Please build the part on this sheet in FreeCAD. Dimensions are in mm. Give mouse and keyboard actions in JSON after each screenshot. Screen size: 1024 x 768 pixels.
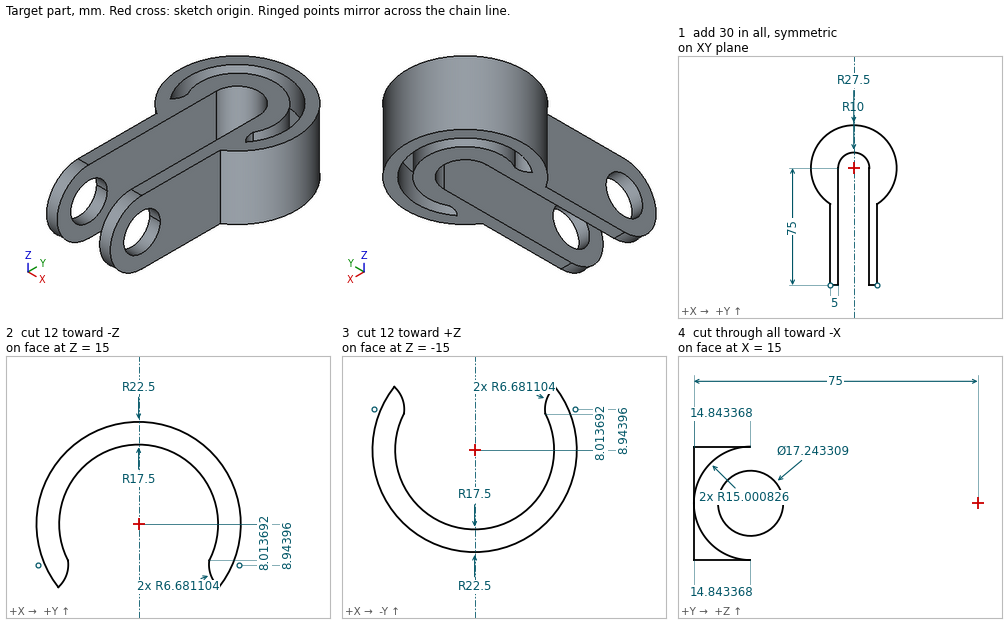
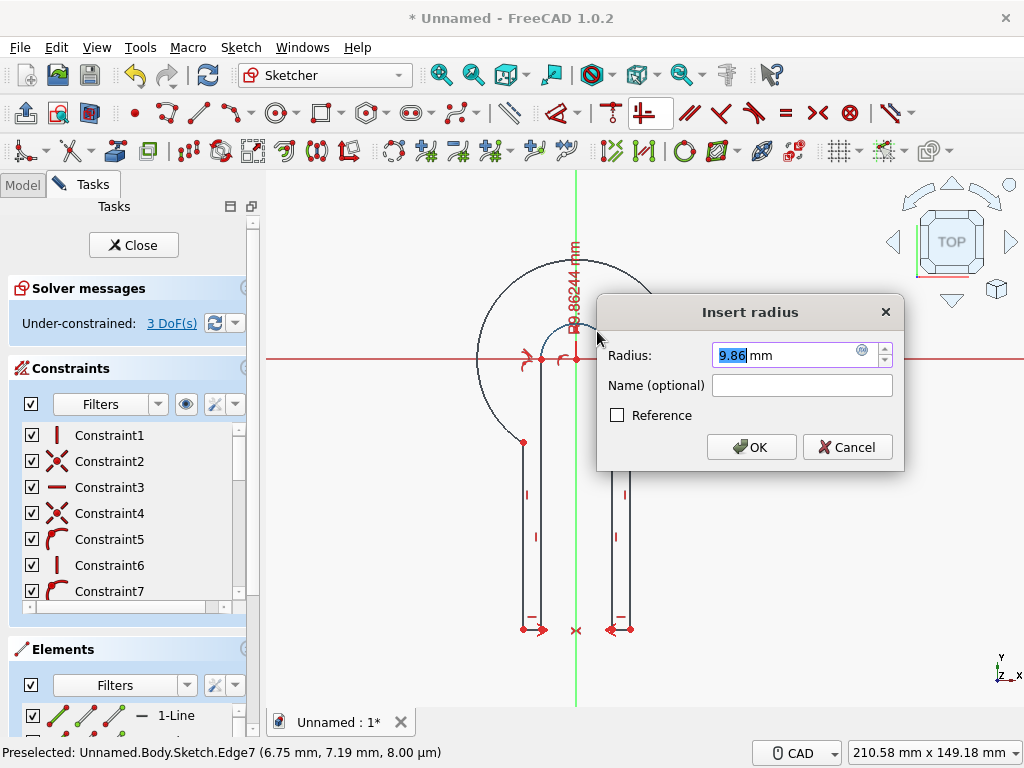
{"action": "type", "text": "10"}
{"action": "key", "text": "Return"}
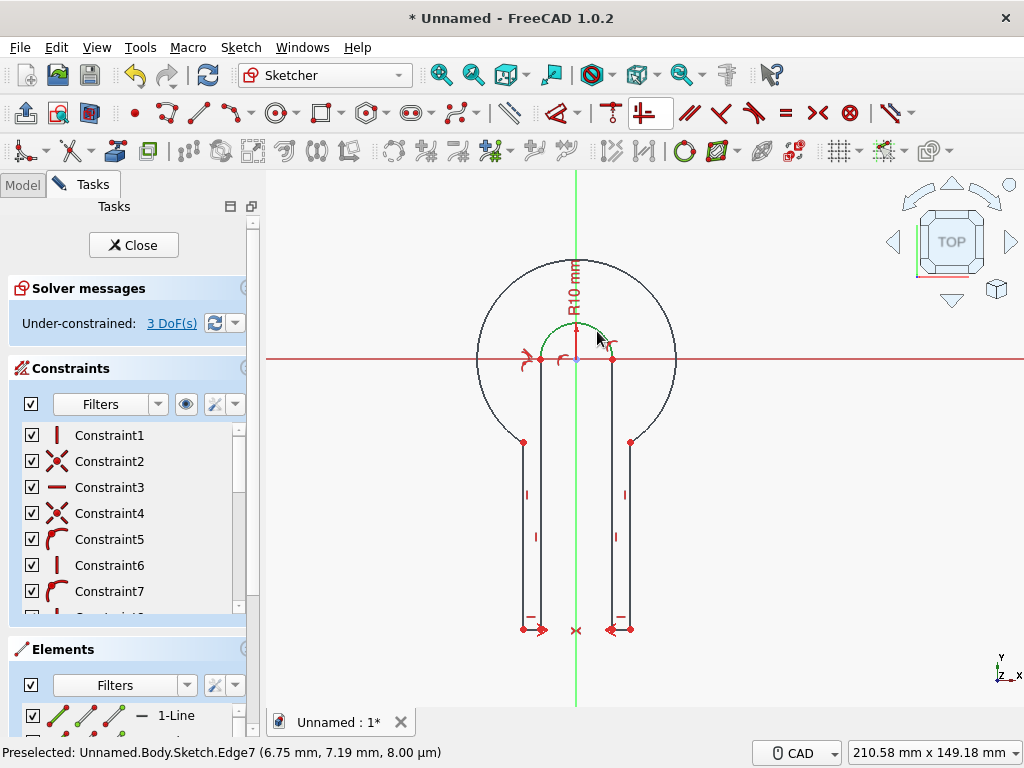
{"action": "left_click", "coordinate": [662, 308]}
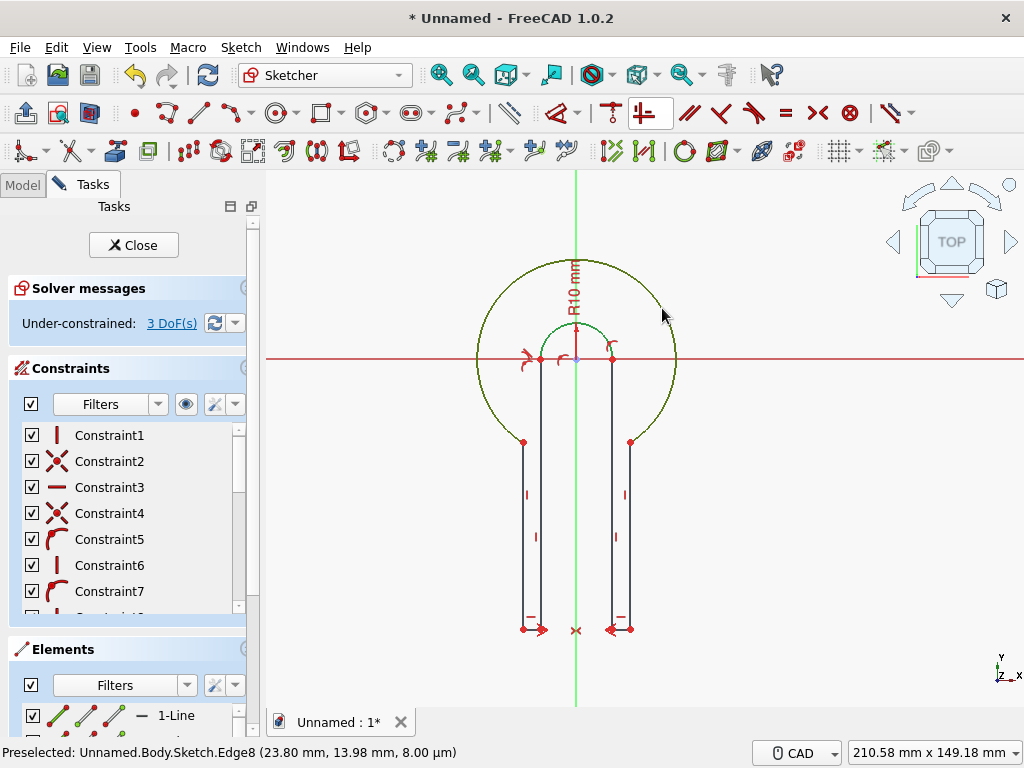
{"action": "key", "text": "k r"}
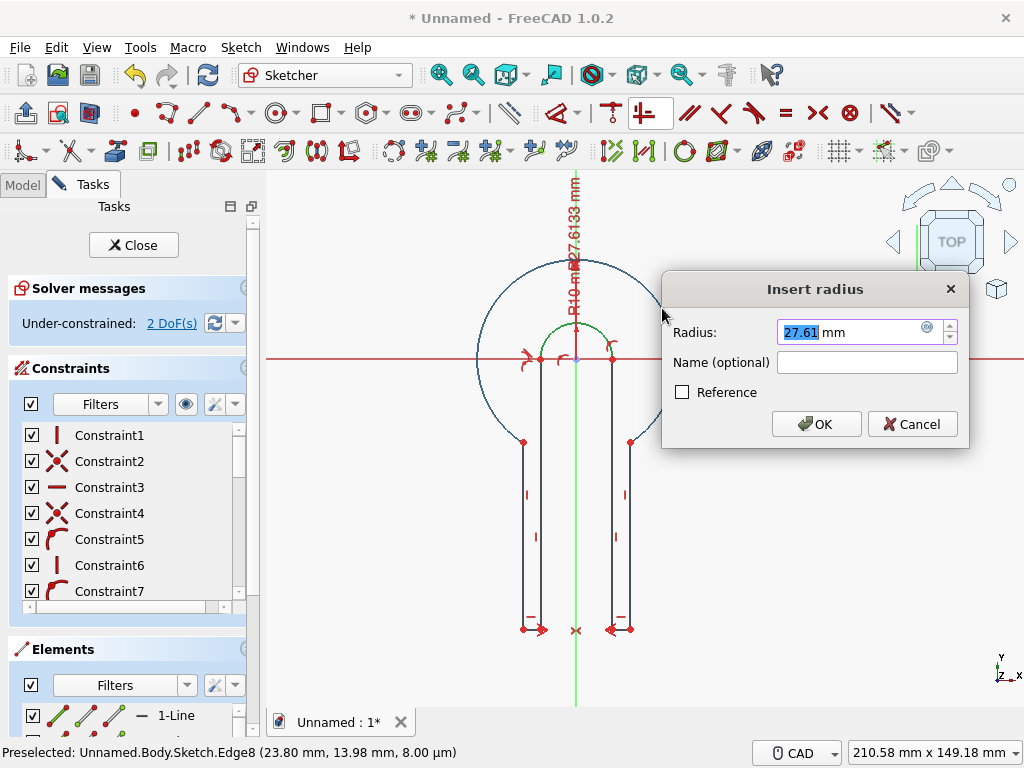
{"action": "type", "text": "27.5"}
{"action": "key", "text": "Return"}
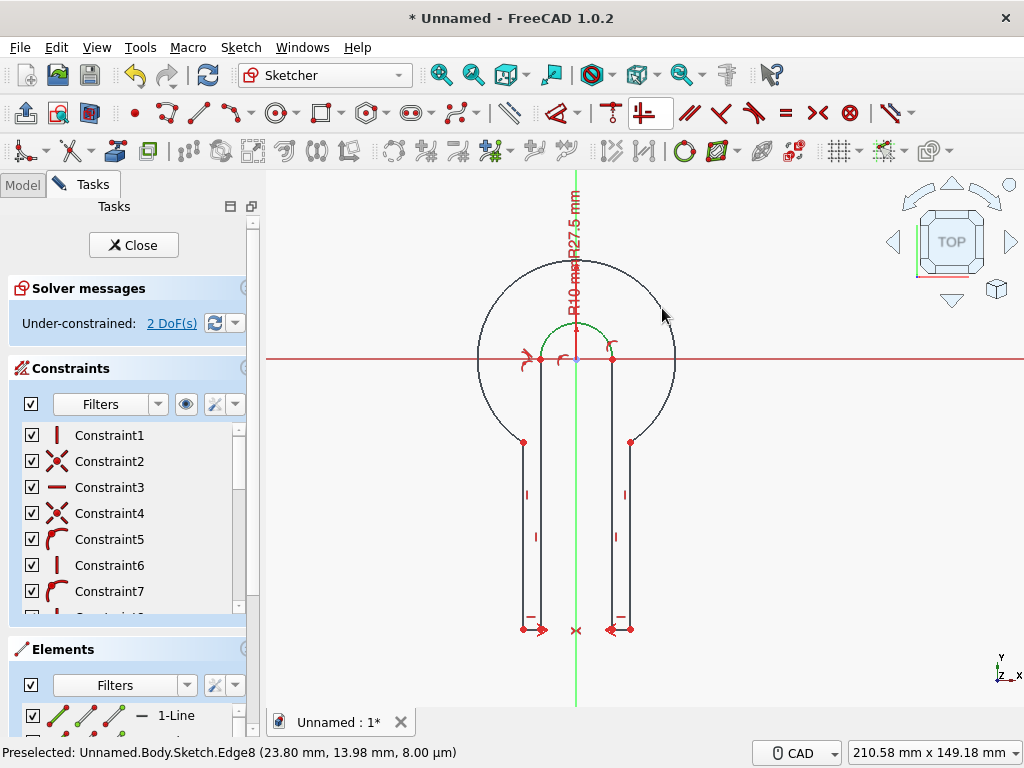
{"action": "scroll", "coordinate": [532, 630], "scroll_direction": "up", "scroll_amount": 4}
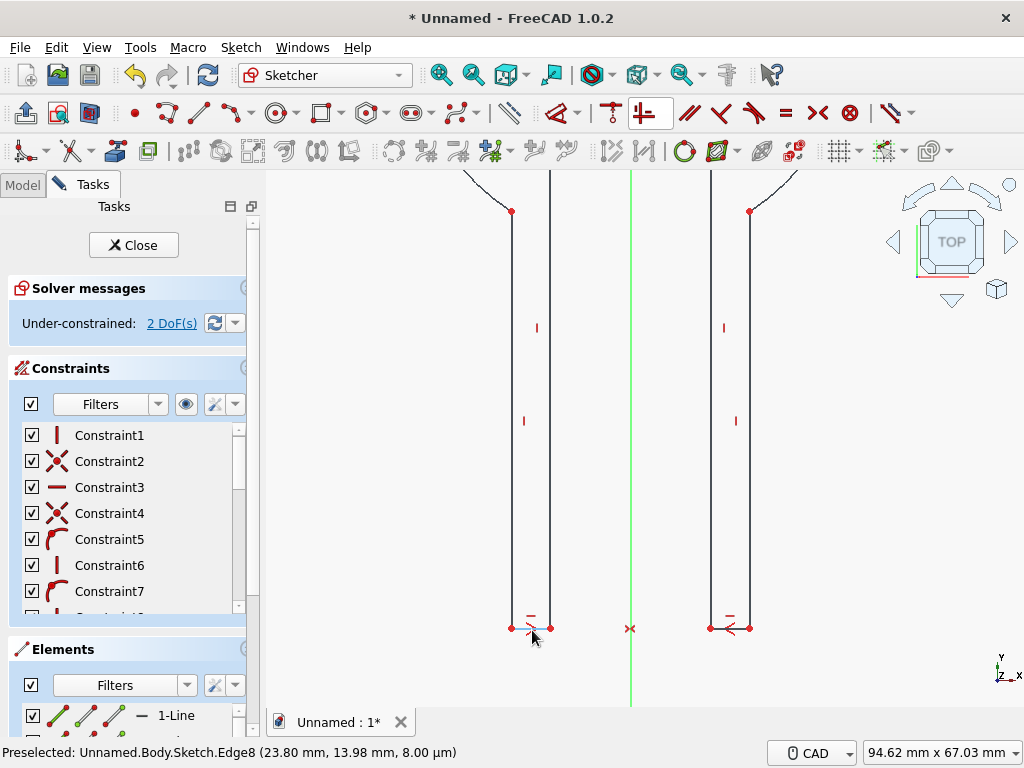
{"action": "left_click", "coordinate": [531, 629]}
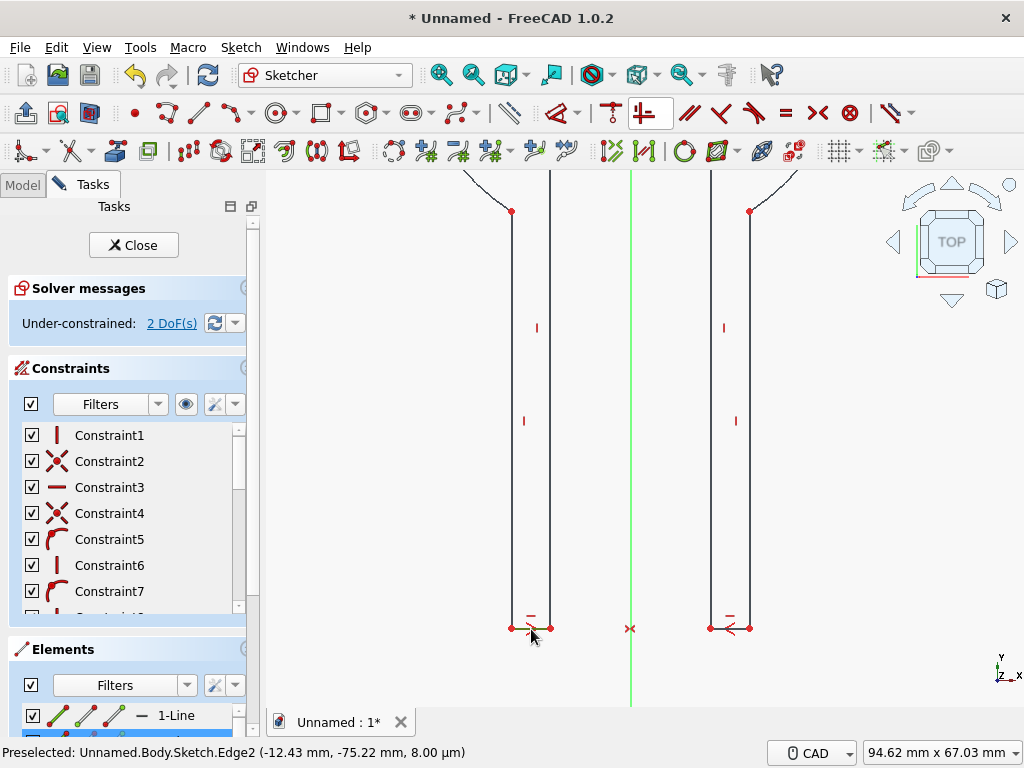
{"action": "left_click", "coordinate": [580, 114]}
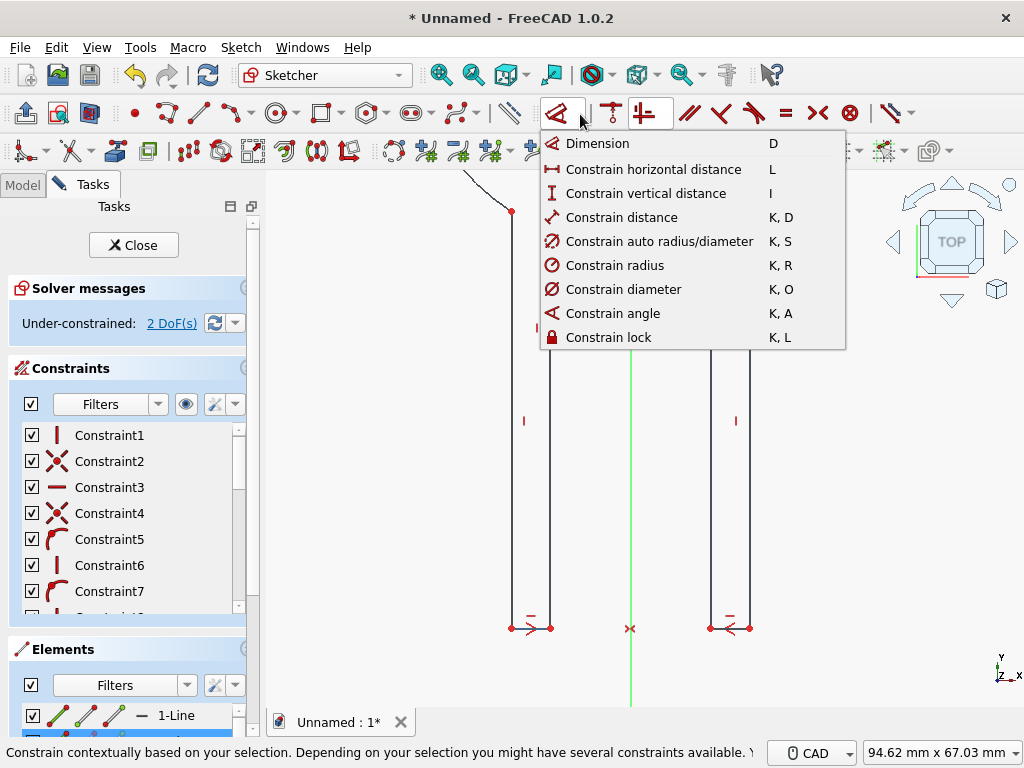
{"action": "left_click", "coordinate": [693, 169]}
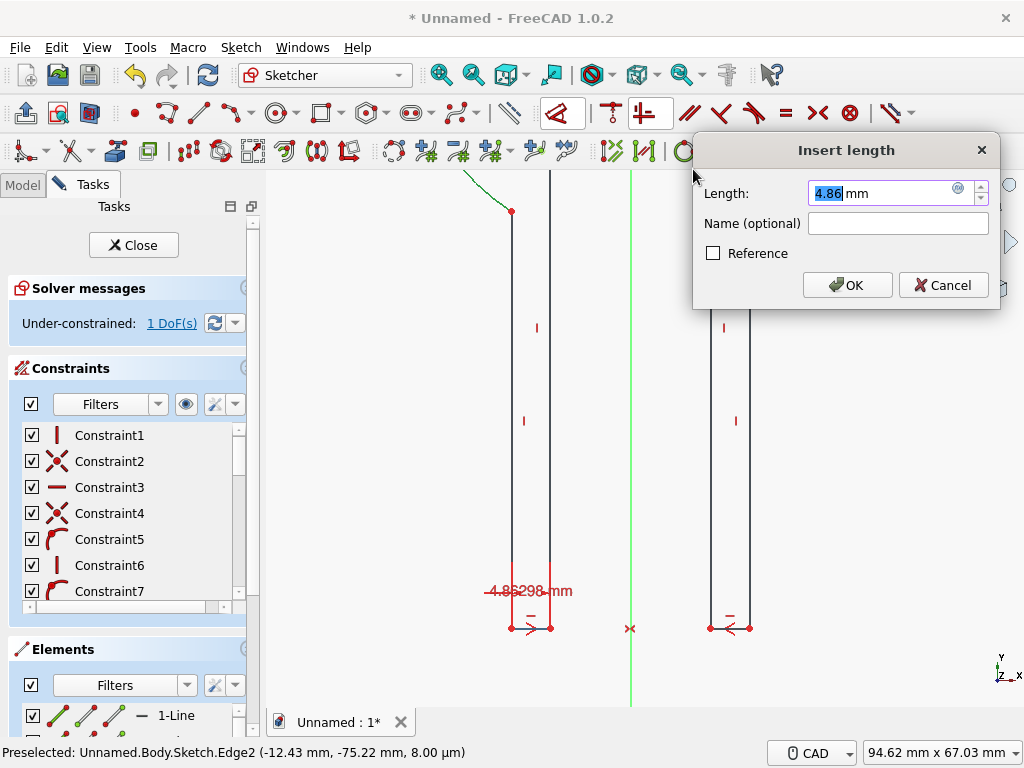
{"action": "type", "text": "5"}
{"action": "key", "text": "Return"}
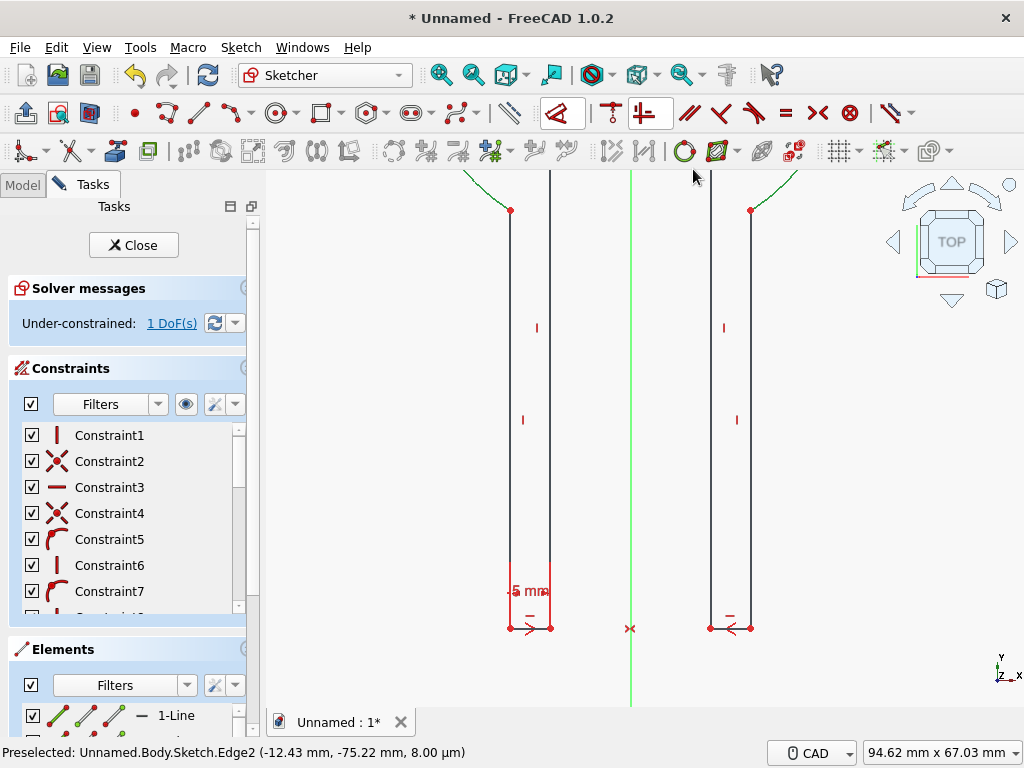
{"action": "left_click", "coordinate": [550, 448]}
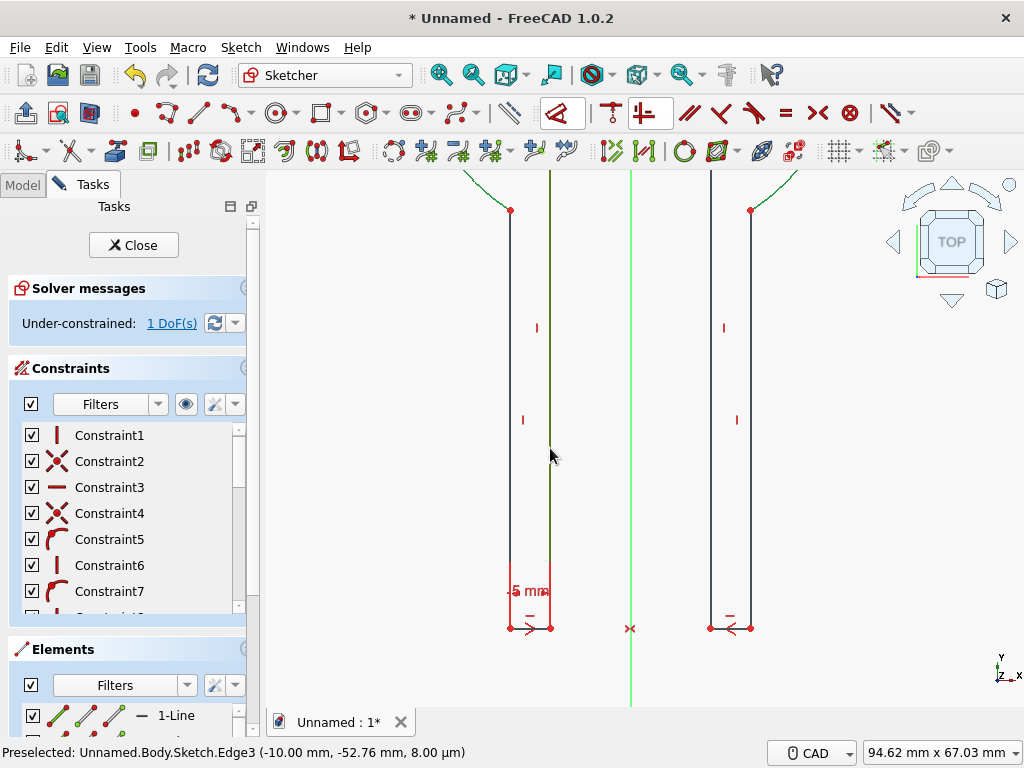
{"action": "key", "text": "i"}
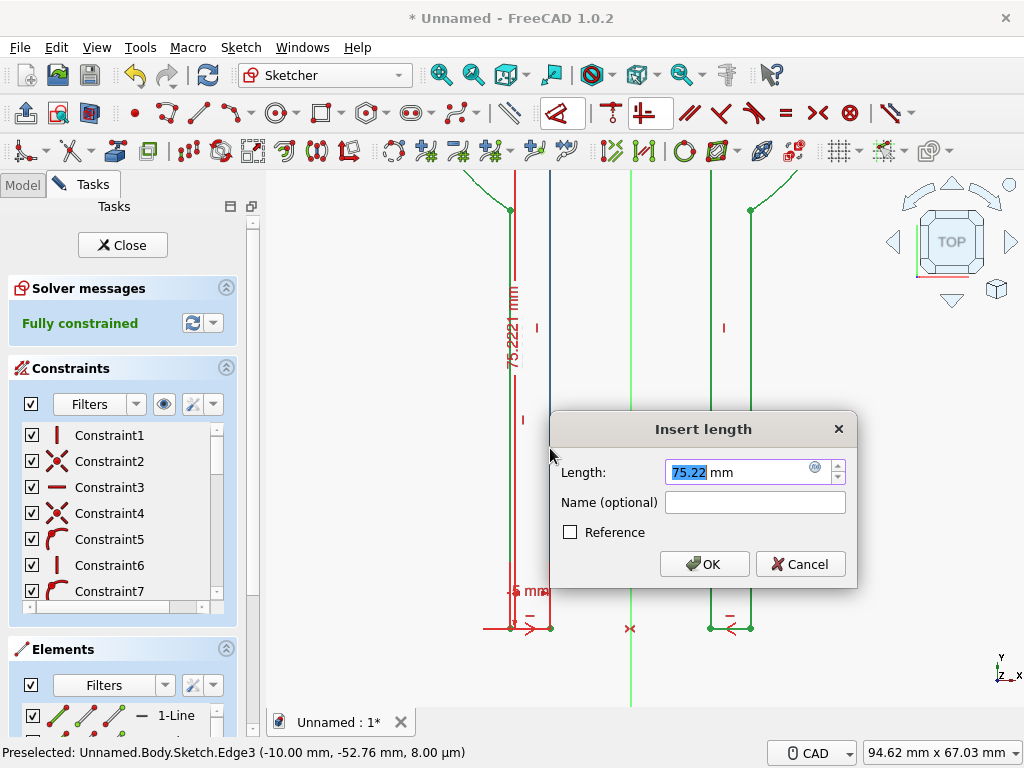
{"action": "type", "text": "75"}
{"action": "key", "text": "Return"}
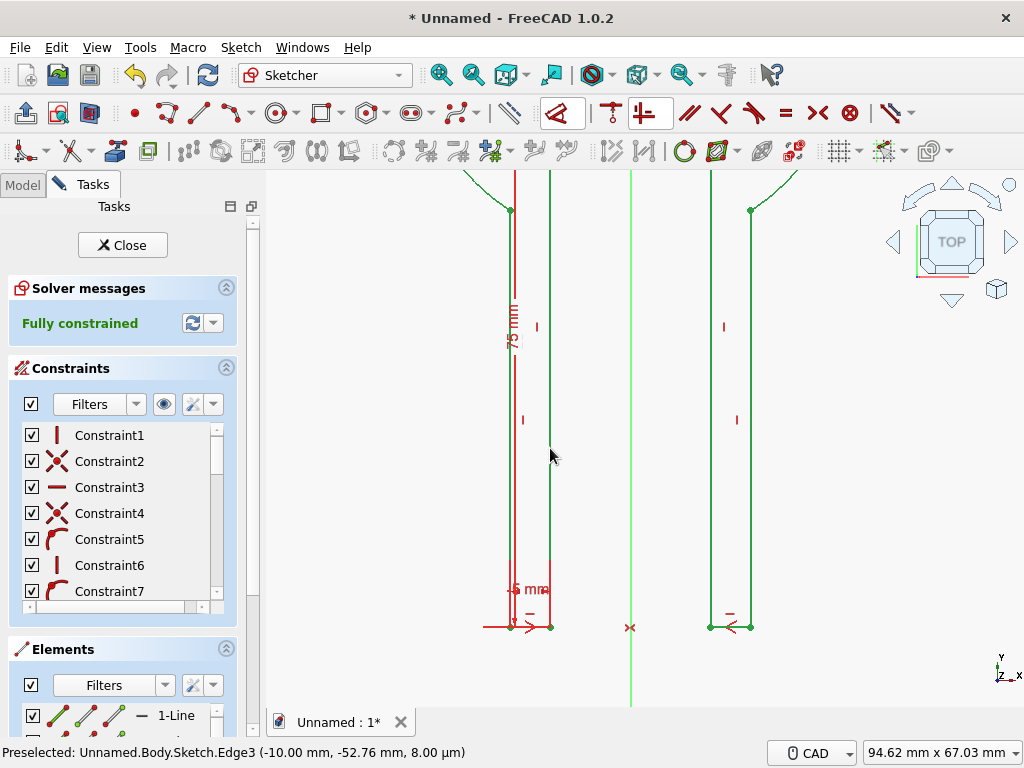
{"action": "left_click", "coordinate": [123, 245]}